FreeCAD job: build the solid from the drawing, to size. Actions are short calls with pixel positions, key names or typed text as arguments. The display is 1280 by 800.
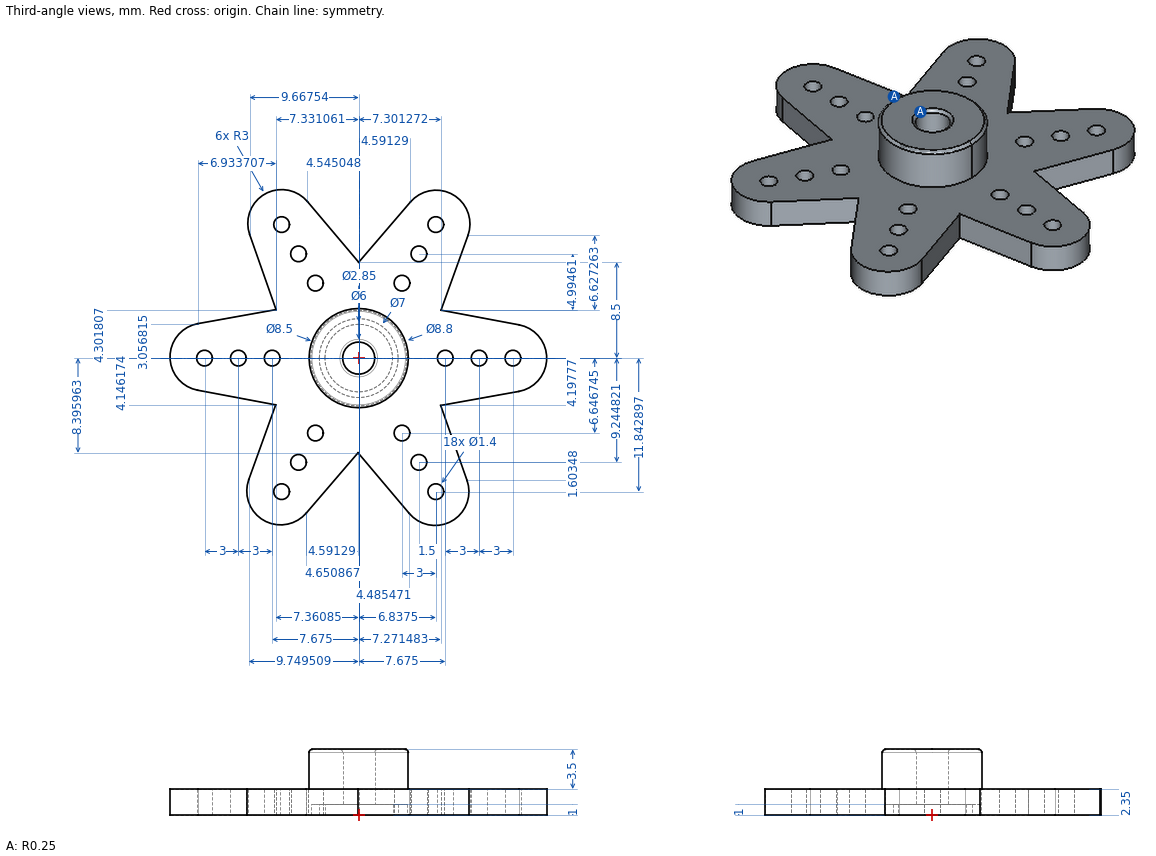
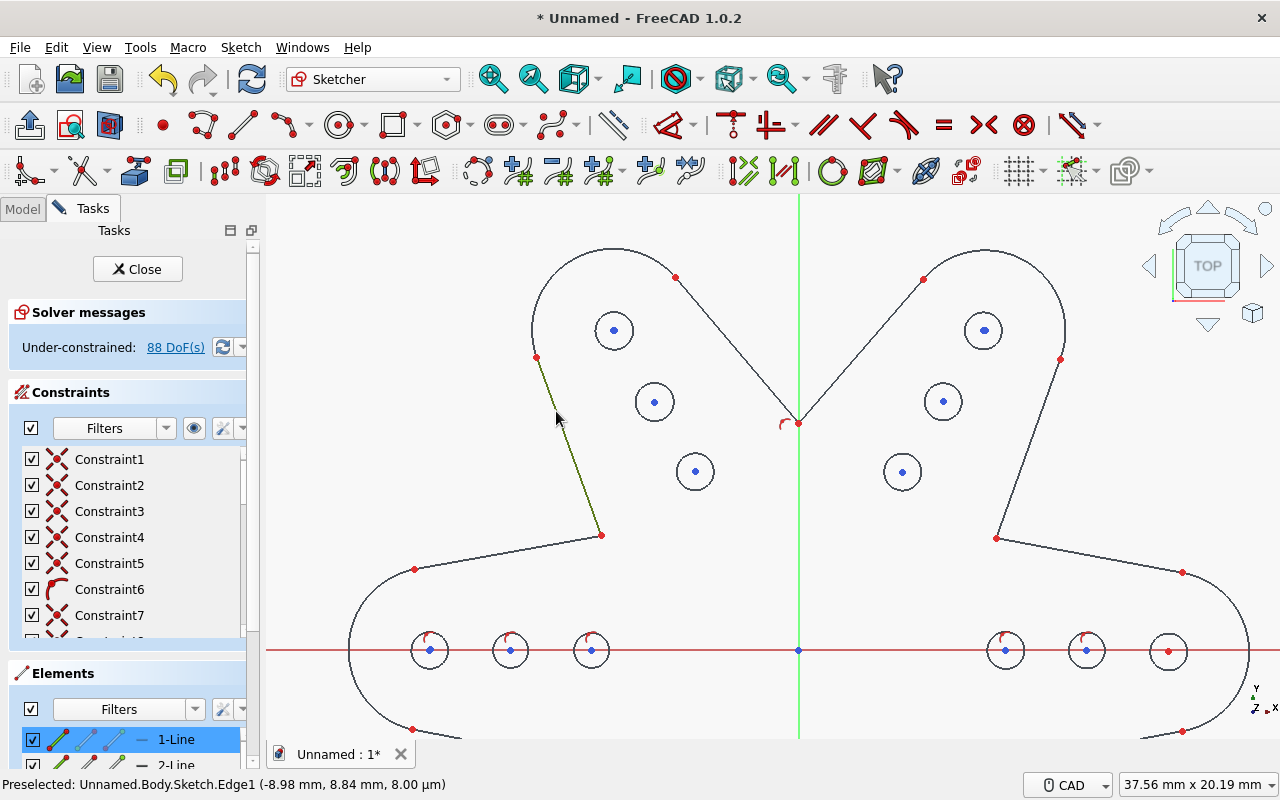
click(616, 249)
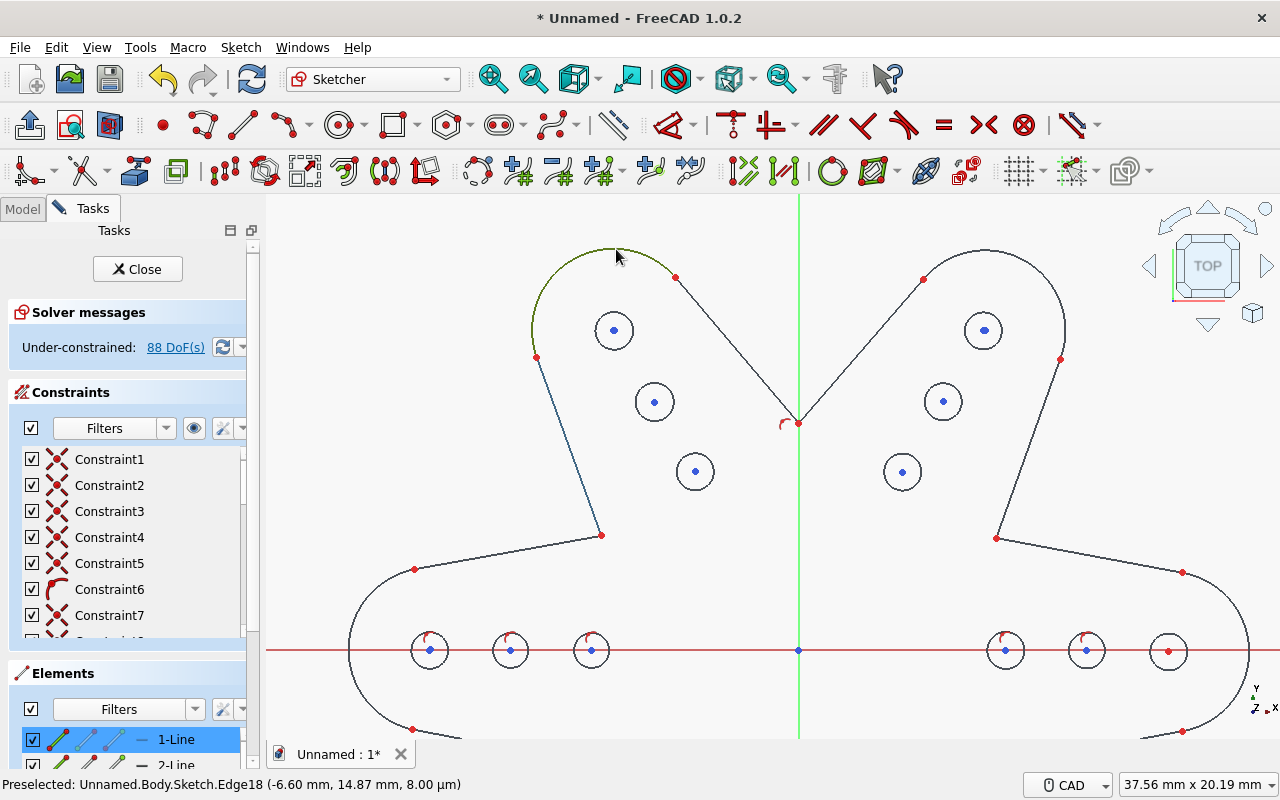
click(904, 126)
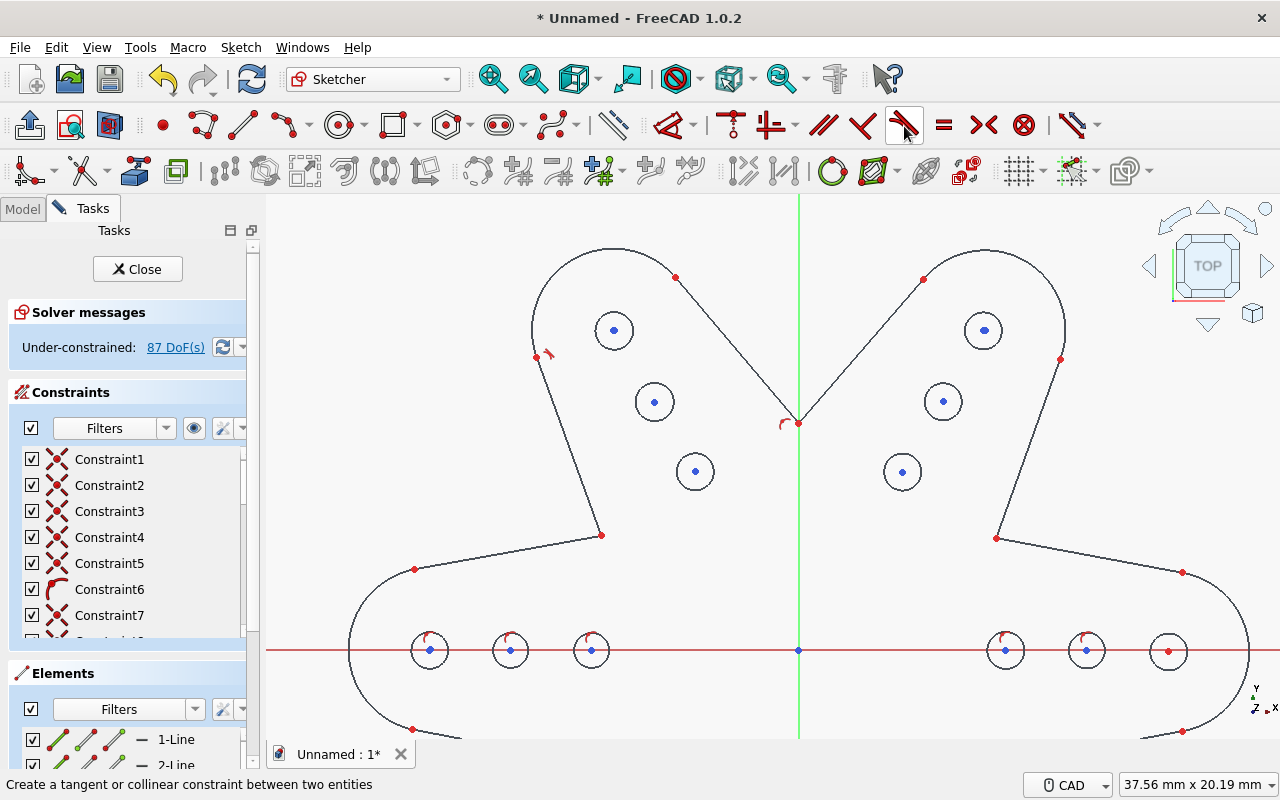
click(545, 546)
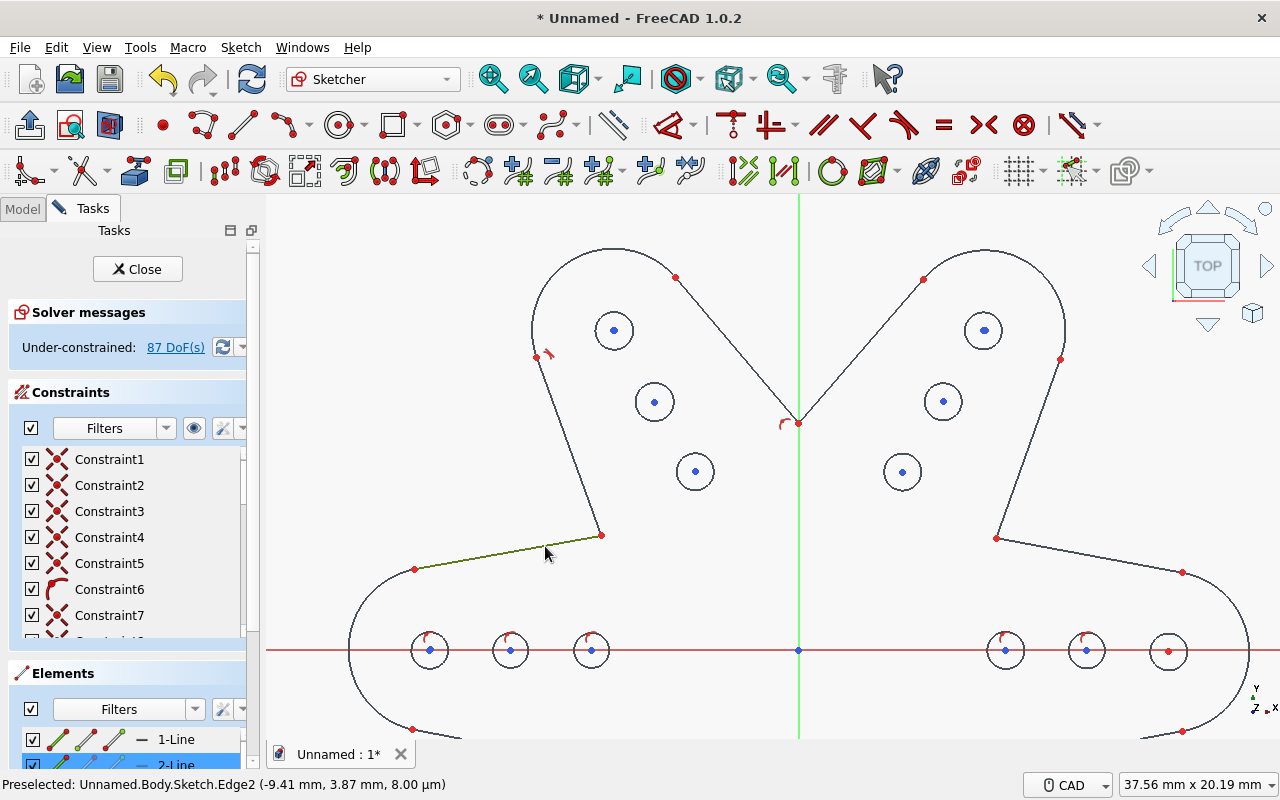
click(361, 606)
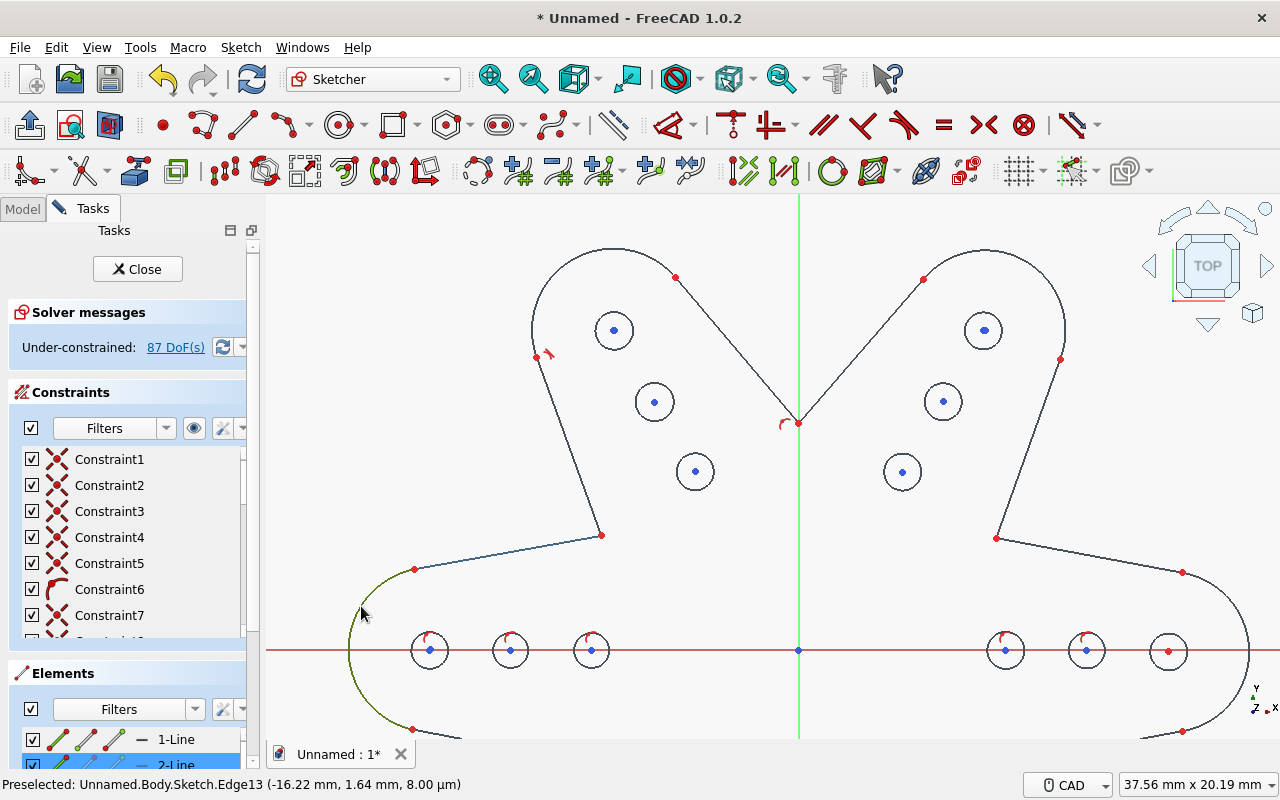
click(904, 126)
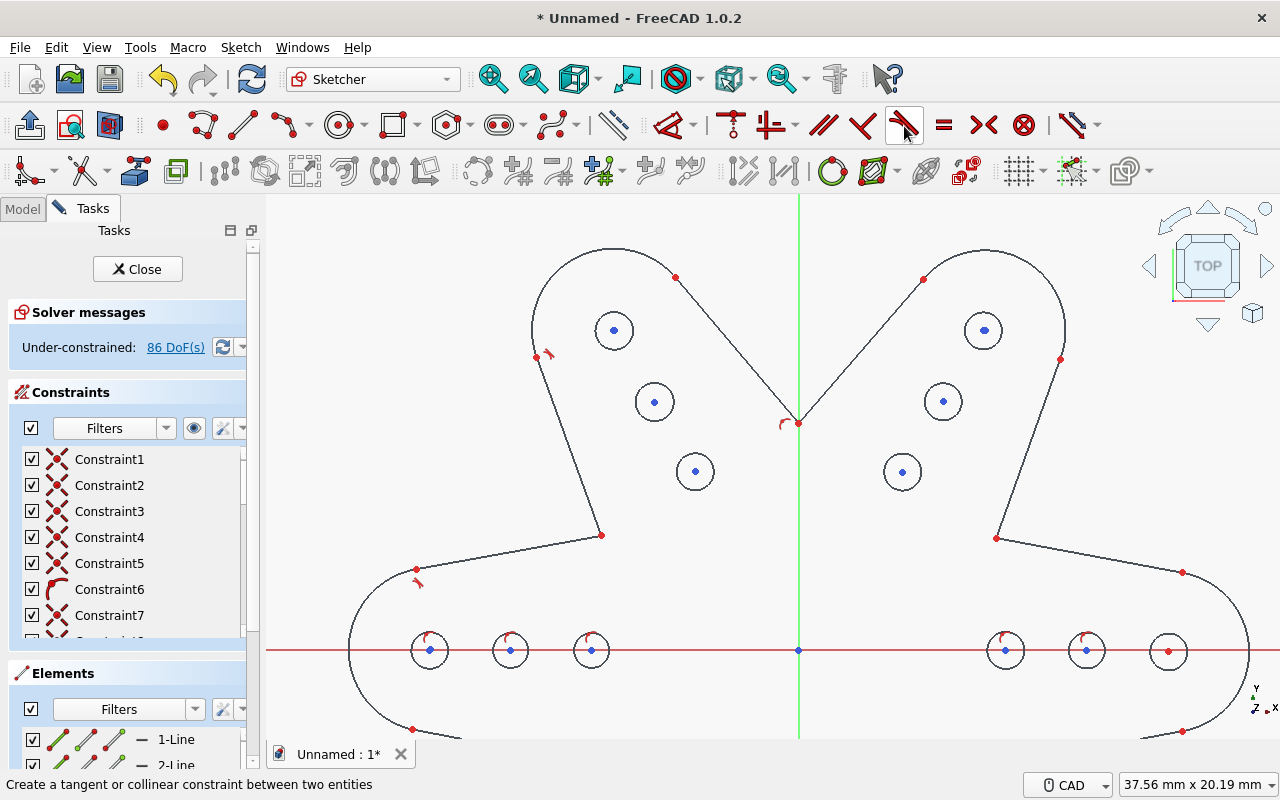
scroll(628, 318, down, 4)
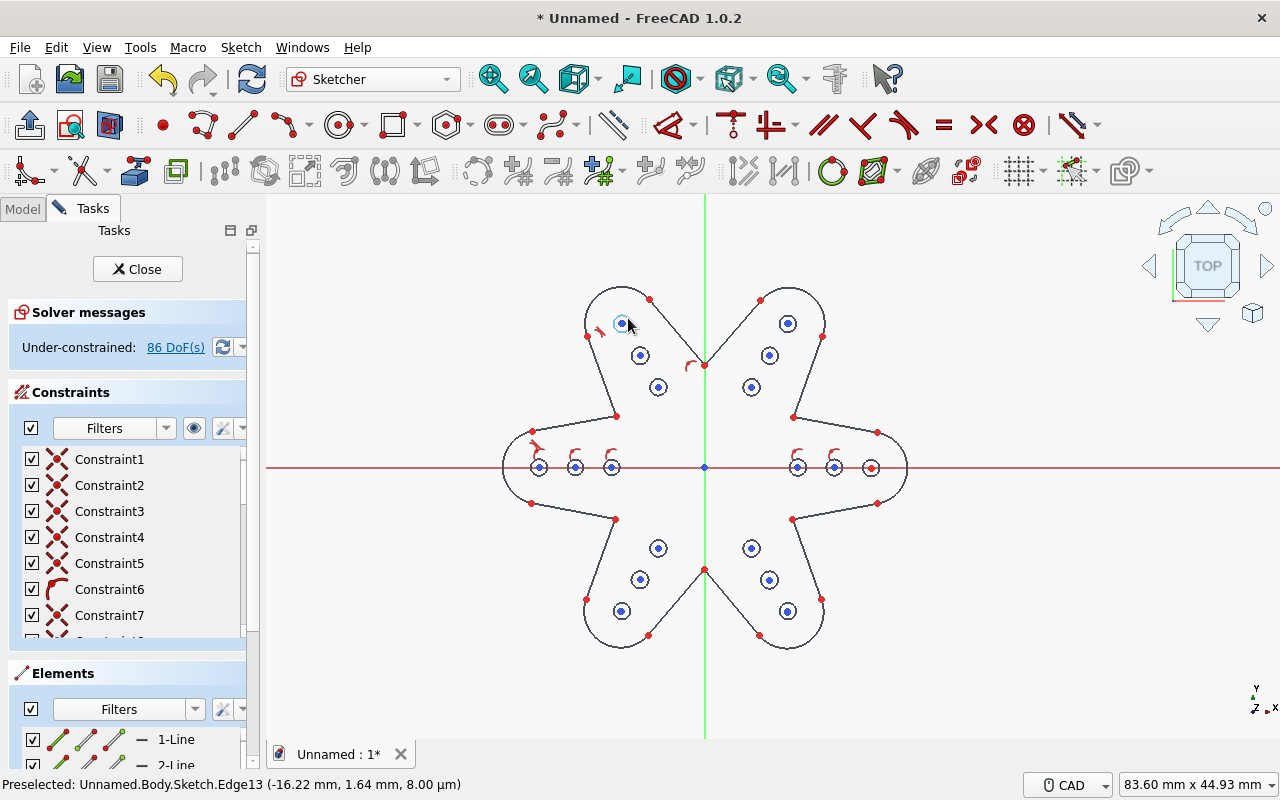
click(556, 508)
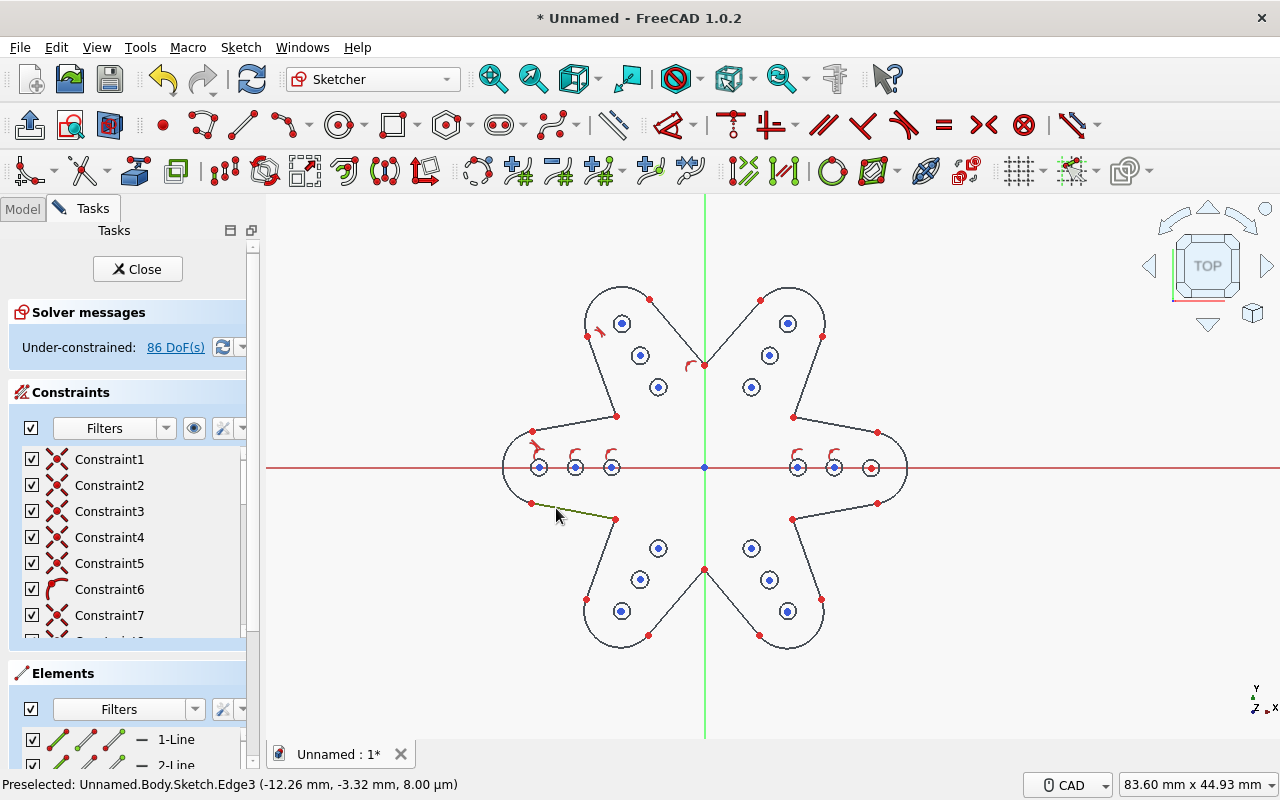
click(509, 447)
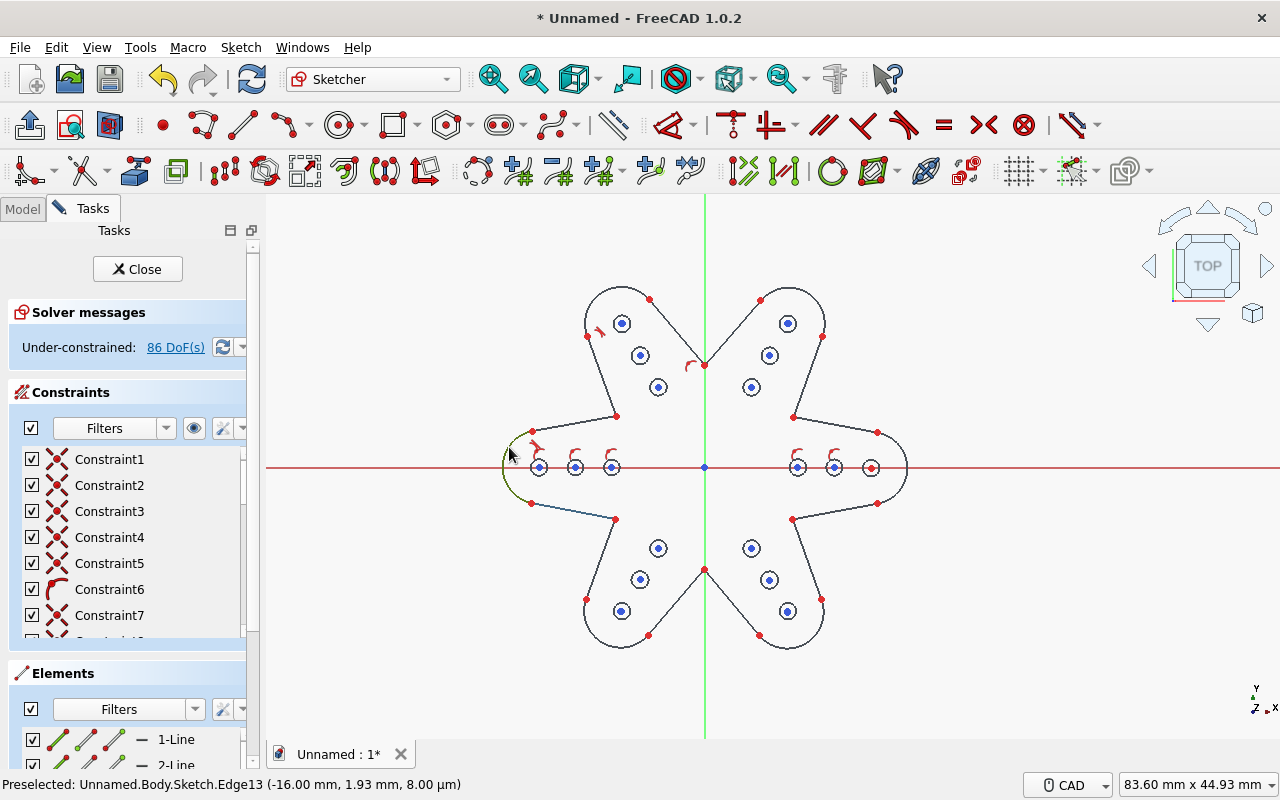
click(904, 126)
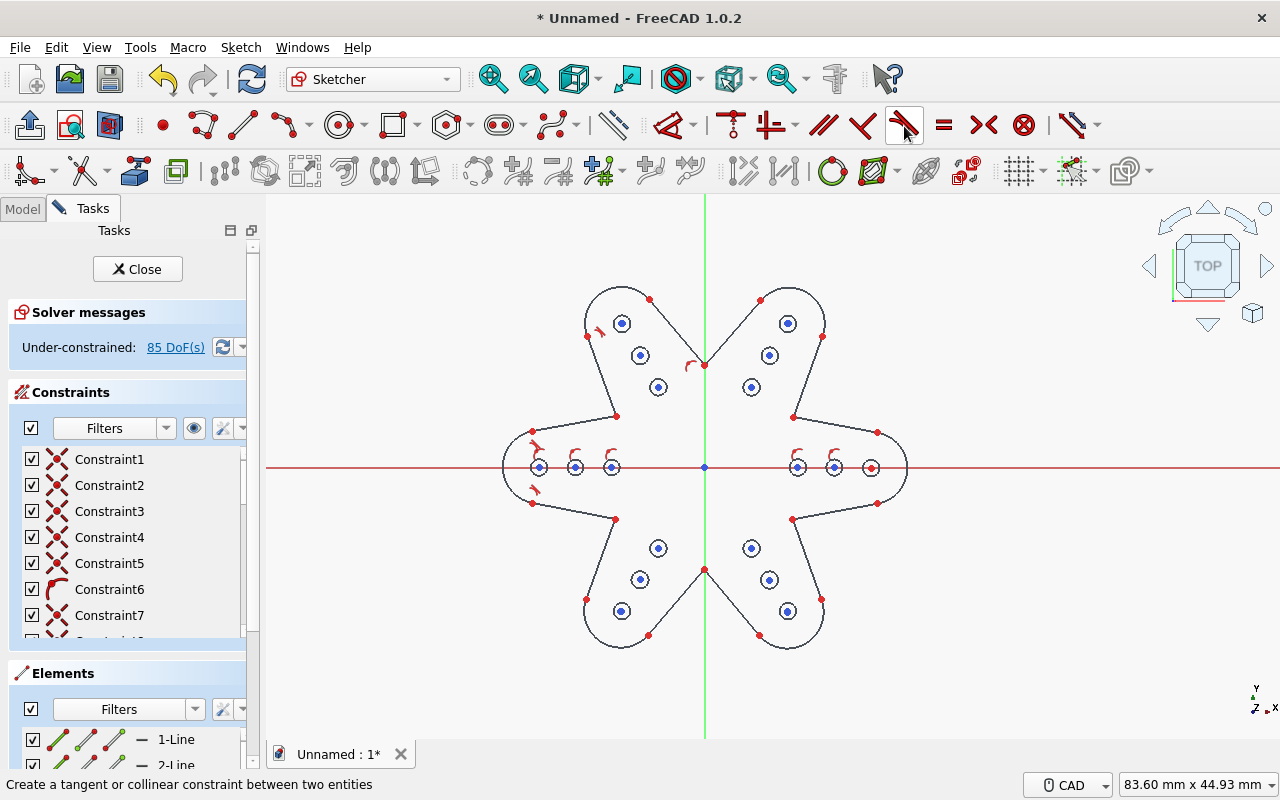
click(607, 543)